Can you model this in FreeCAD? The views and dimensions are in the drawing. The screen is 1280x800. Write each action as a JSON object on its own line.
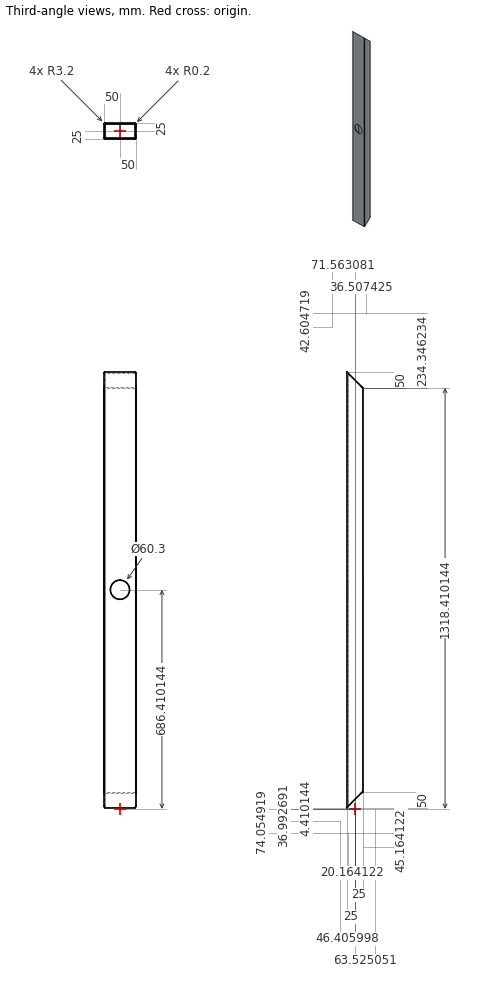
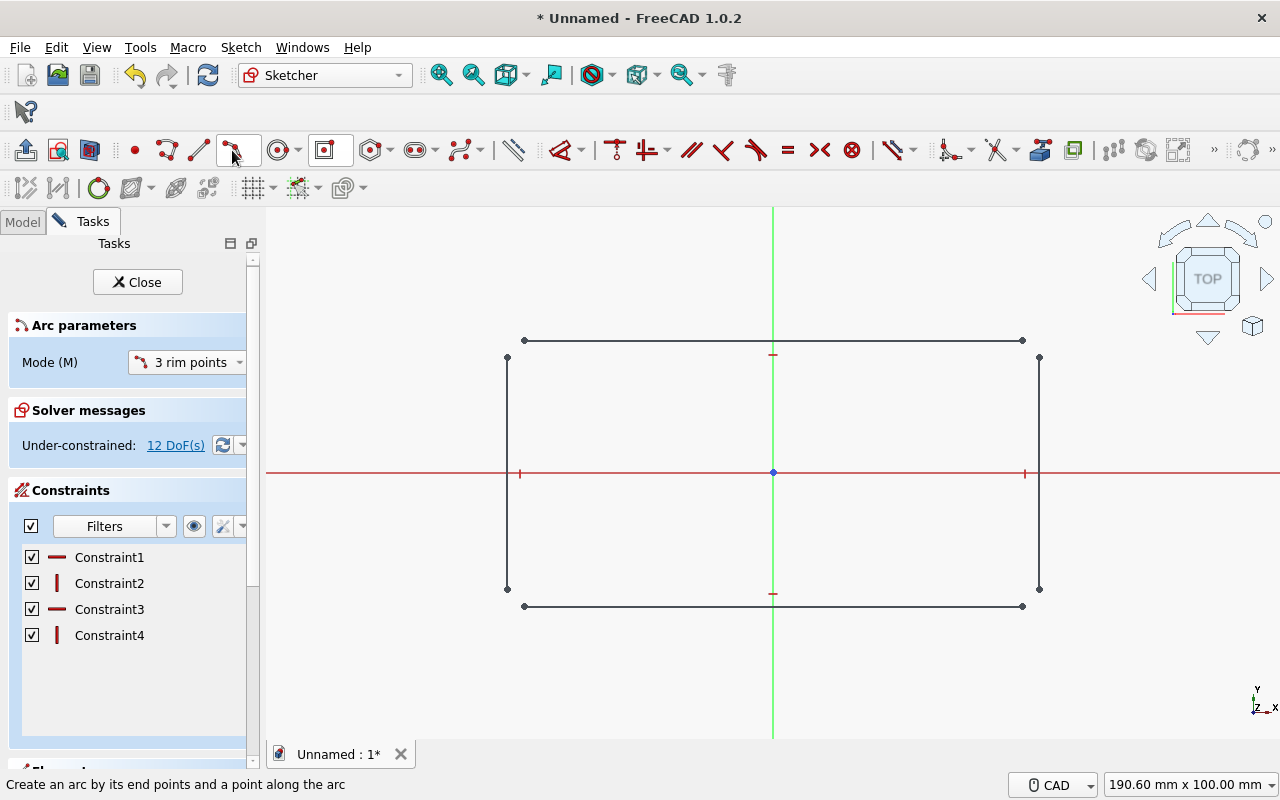
{"action": "left_click", "coordinate": [524, 341]}
{"action": "left_click", "coordinate": [507, 358]}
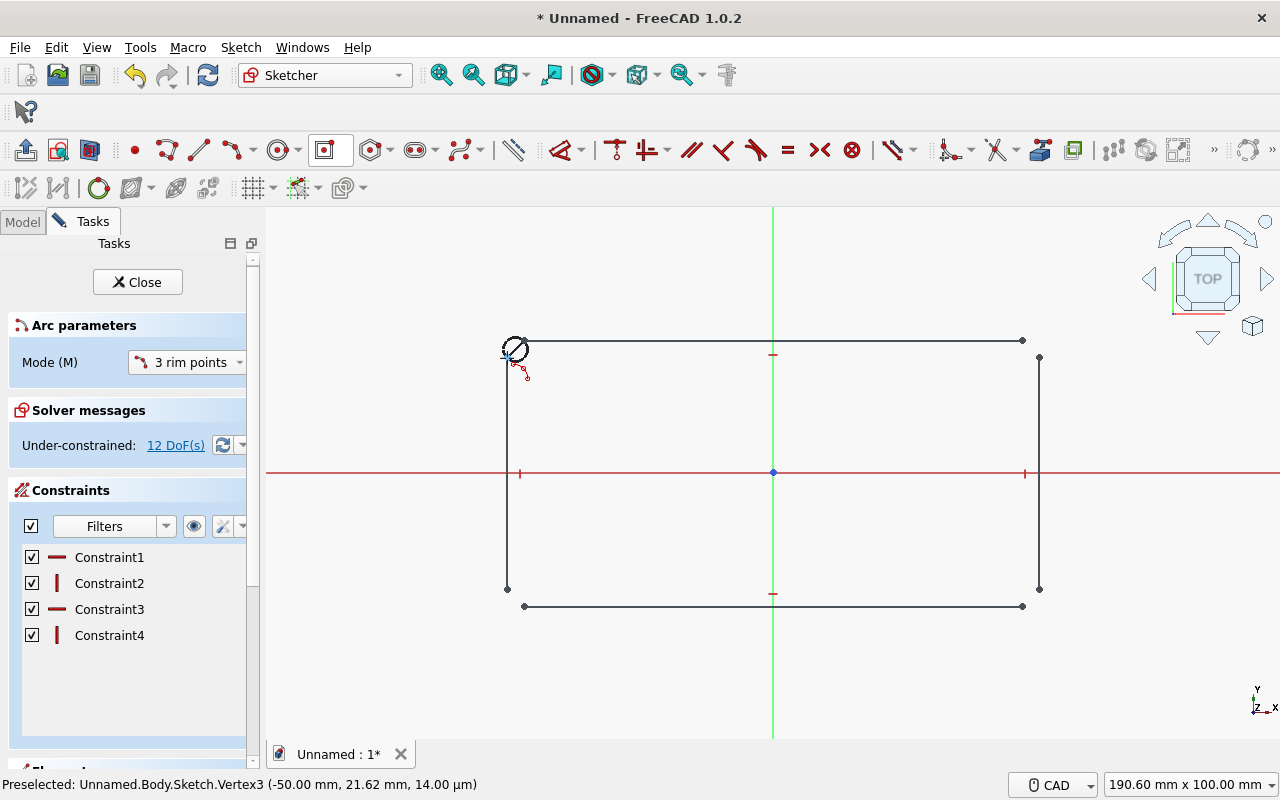
{"action": "scroll", "coordinate": [512, 345], "scroll_direction": "up", "scroll_amount": 6}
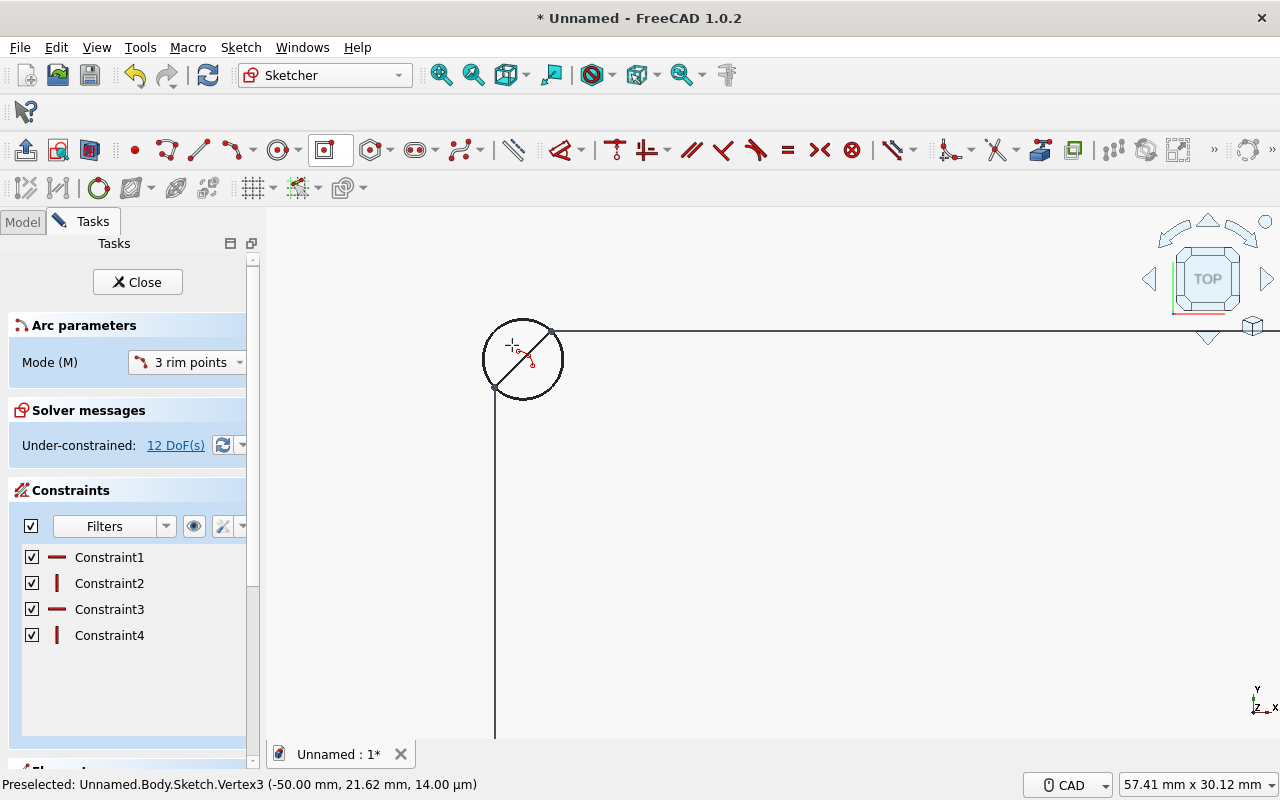
{"action": "left_click", "coordinate": [511, 344]}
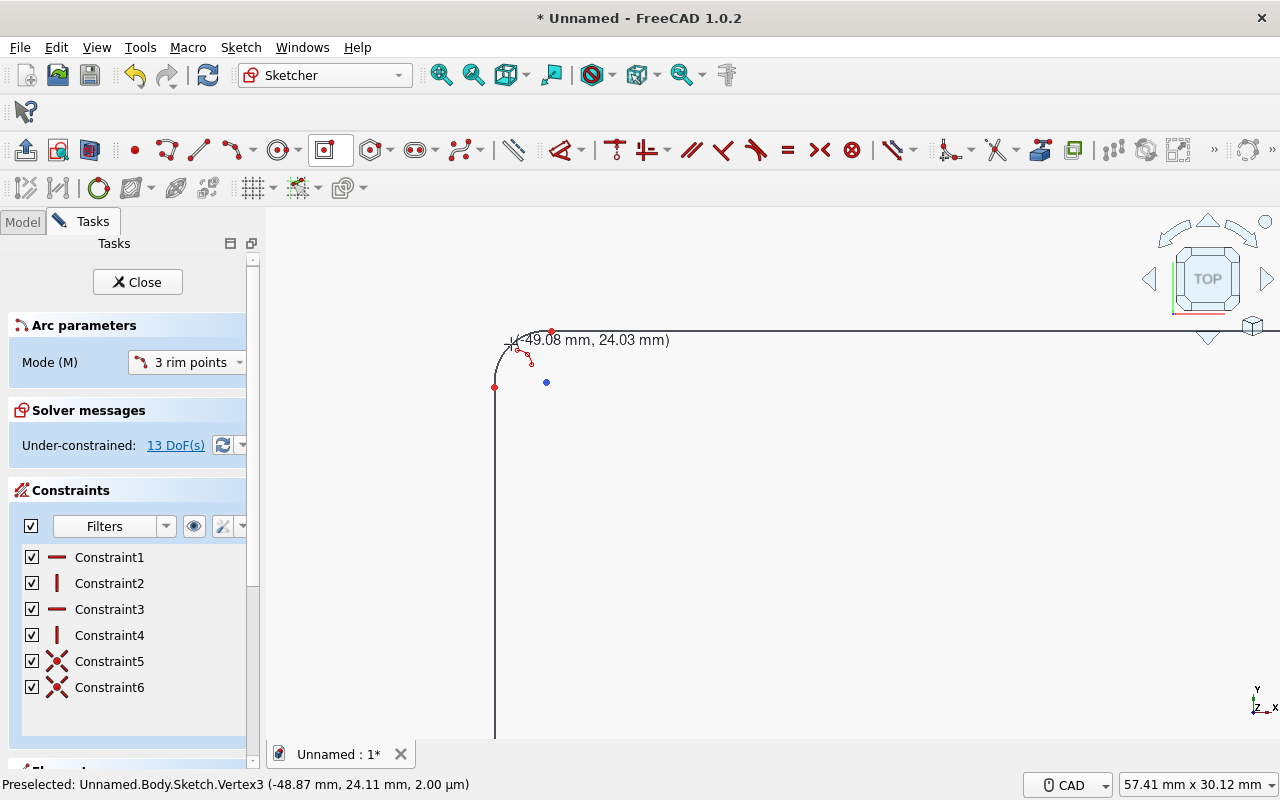
{"action": "scroll", "coordinate": [414, 345], "scroll_direction": "down", "scroll_amount": 6}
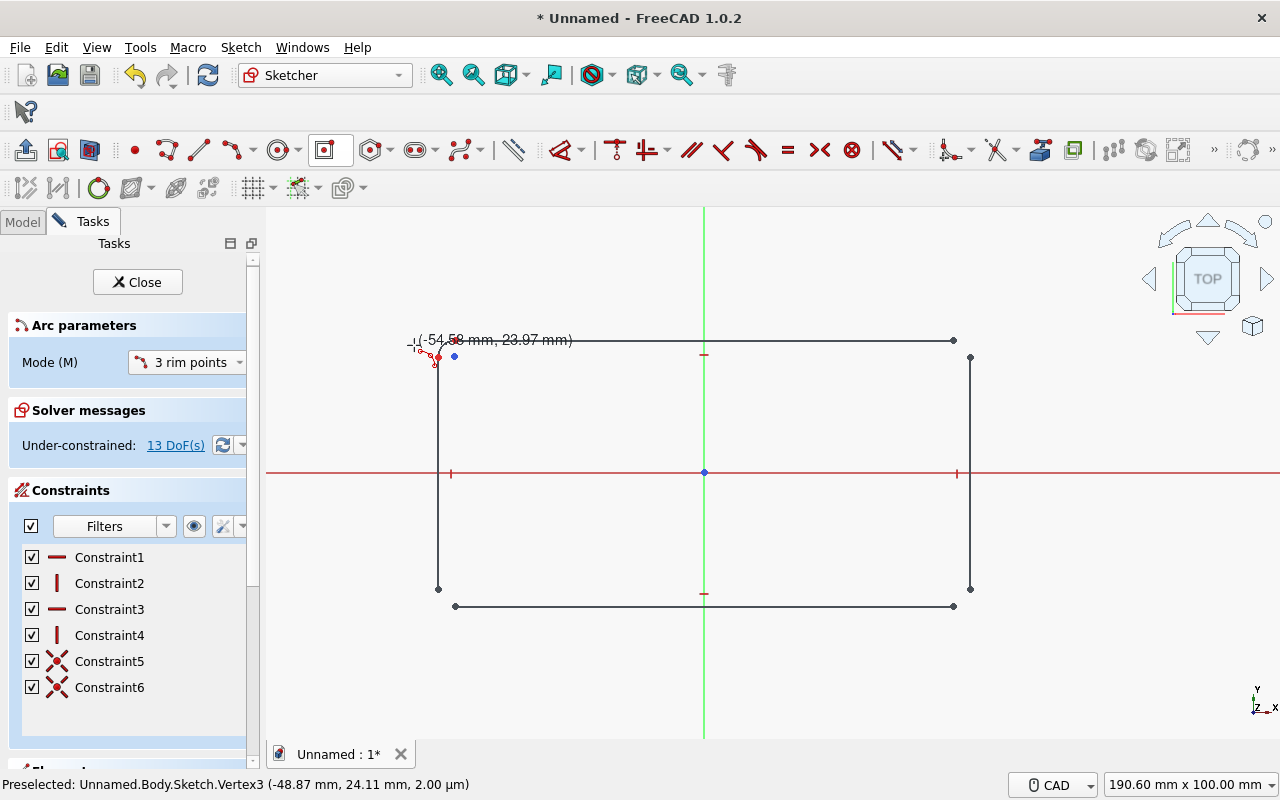
{"action": "left_click", "coordinate": [438, 590]}
{"action": "left_click", "coordinate": [455, 607]}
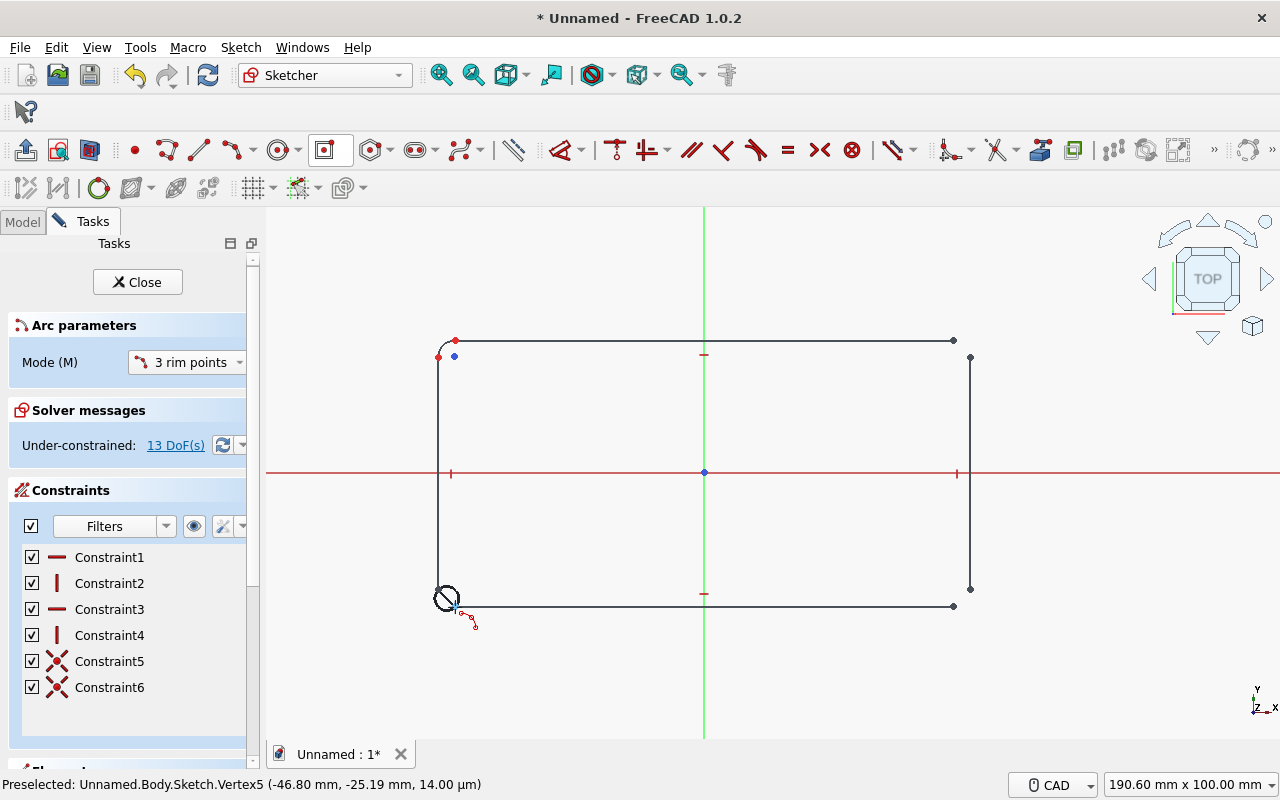
{"action": "scroll", "coordinate": [443, 601], "scroll_direction": "up", "scroll_amount": 6}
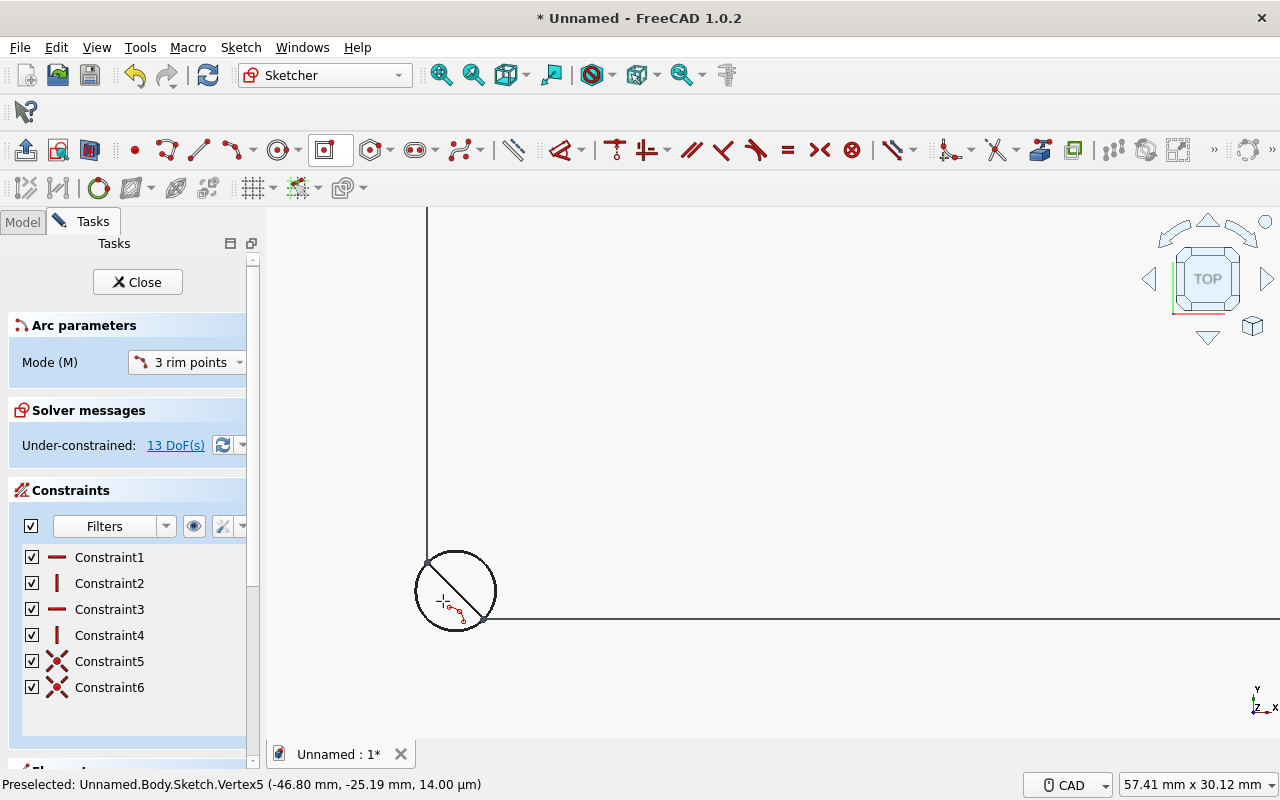
{"action": "left_click", "coordinate": [444, 599]}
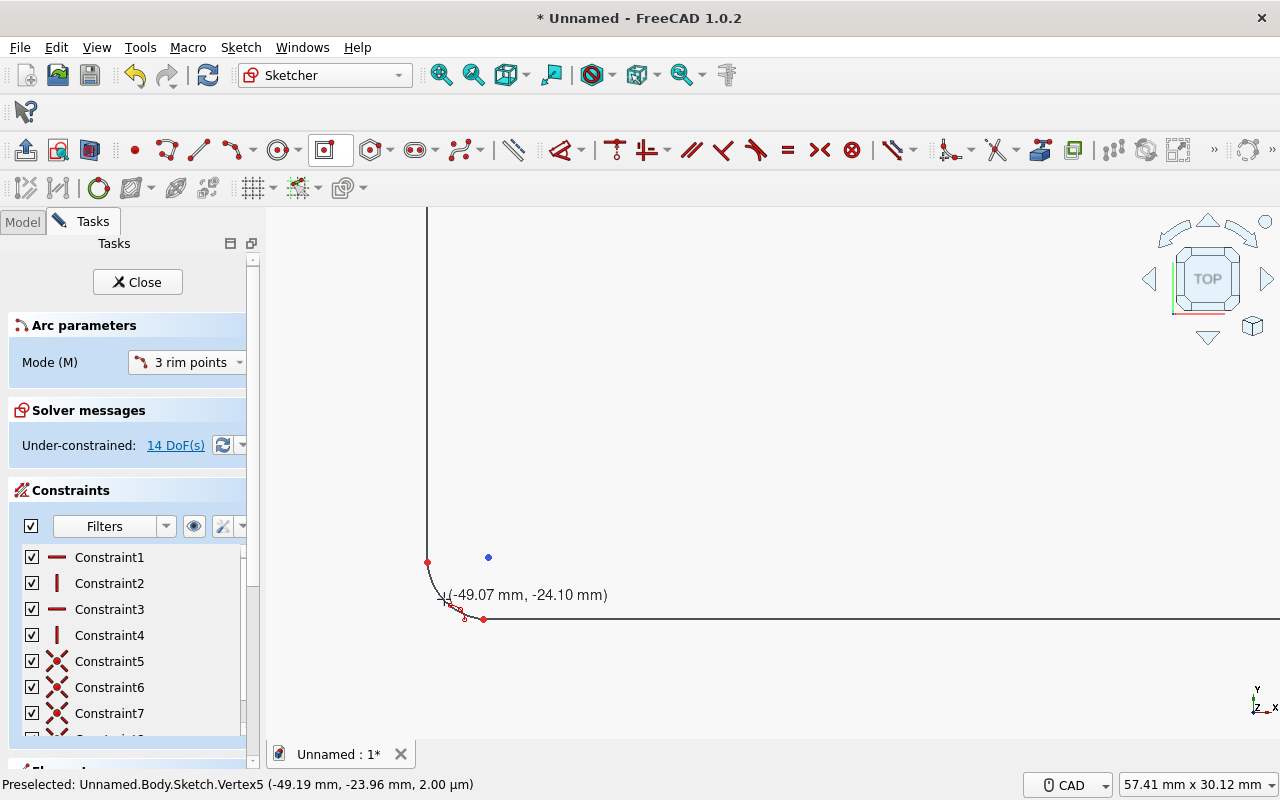
{"action": "scroll", "coordinate": [443, 602], "scroll_direction": "down", "scroll_amount": 6}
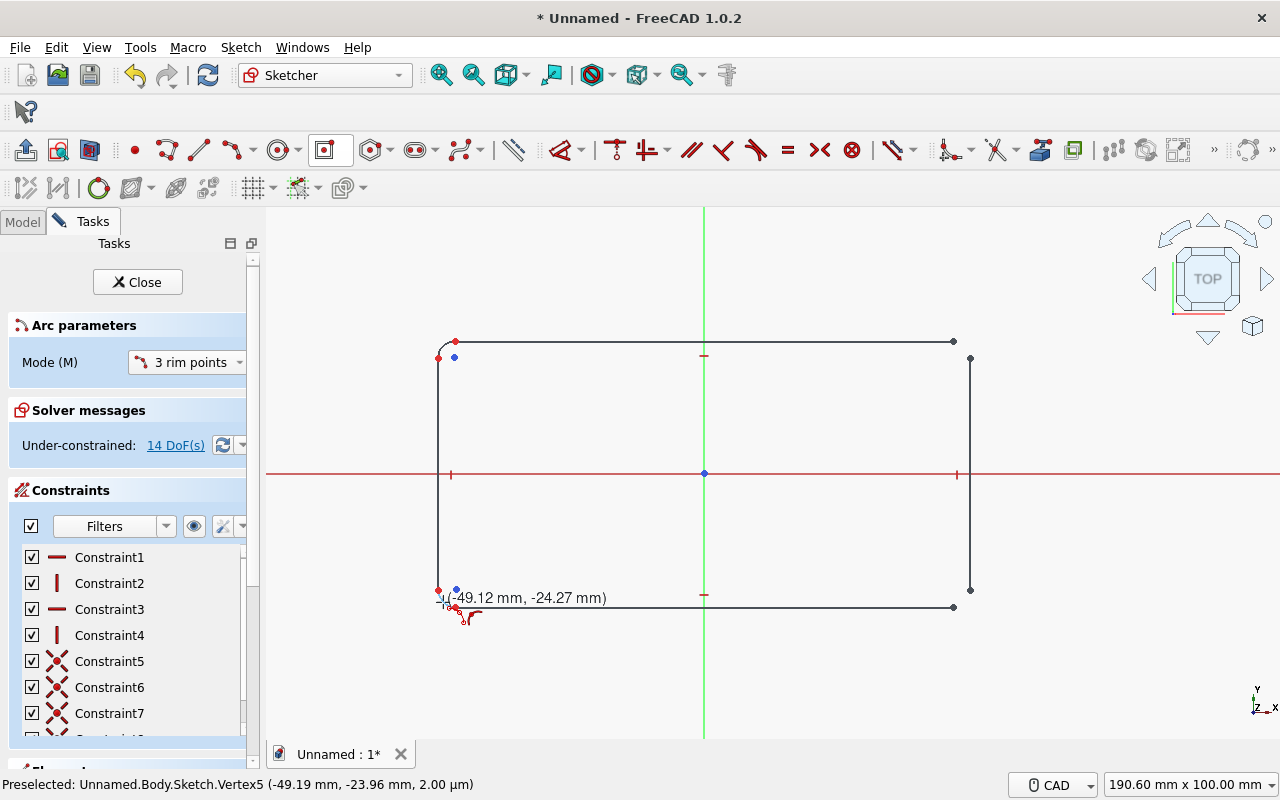
{"action": "left_click", "coordinate": [953, 608]}
{"action": "left_click", "coordinate": [970, 591]}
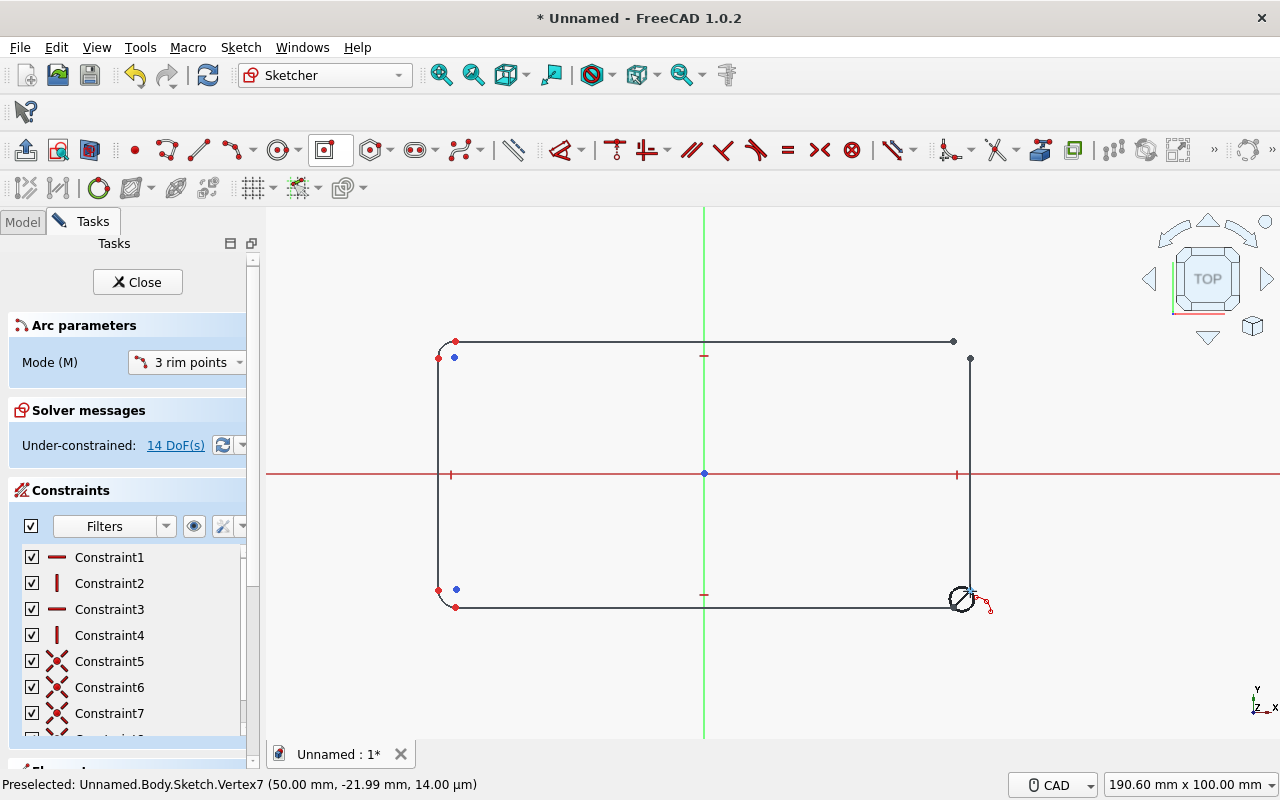
{"action": "scroll", "coordinate": [965, 602], "scroll_direction": "up", "scroll_amount": 6}